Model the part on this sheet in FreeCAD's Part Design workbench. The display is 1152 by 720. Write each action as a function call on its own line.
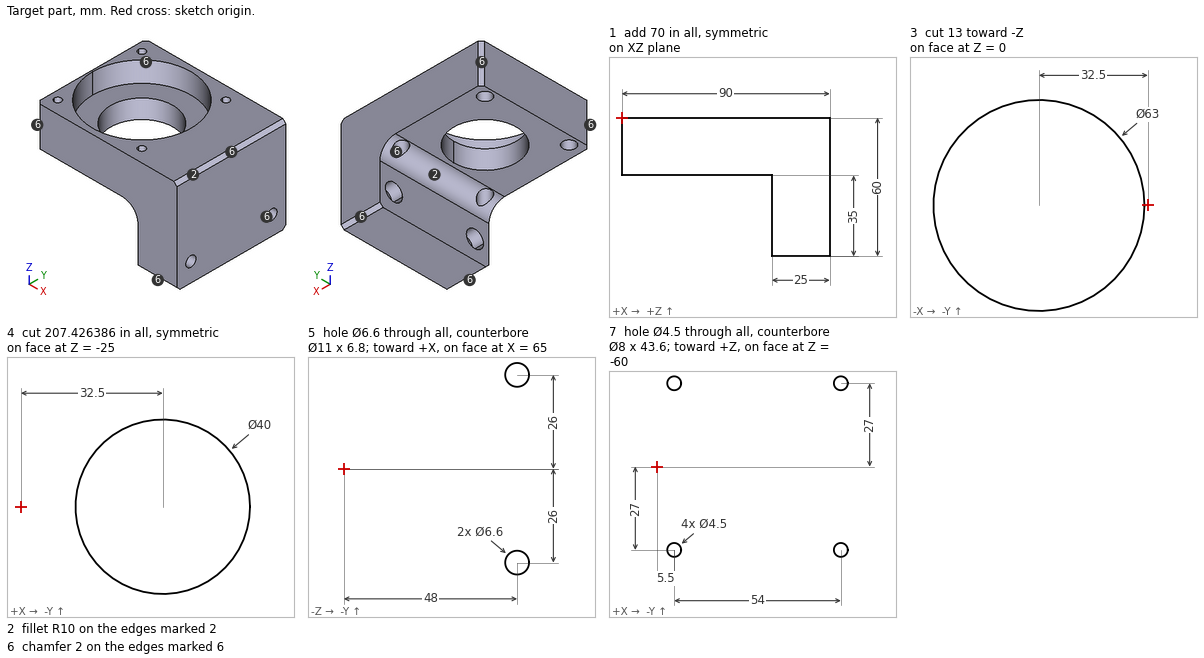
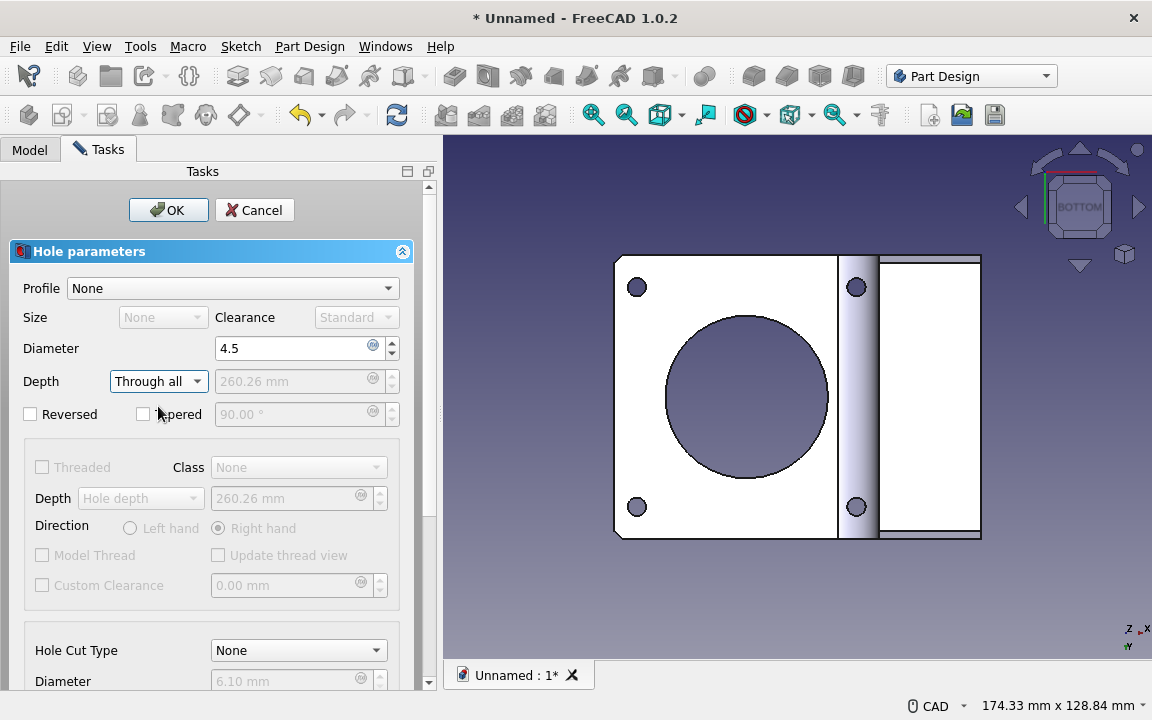
click(300, 650)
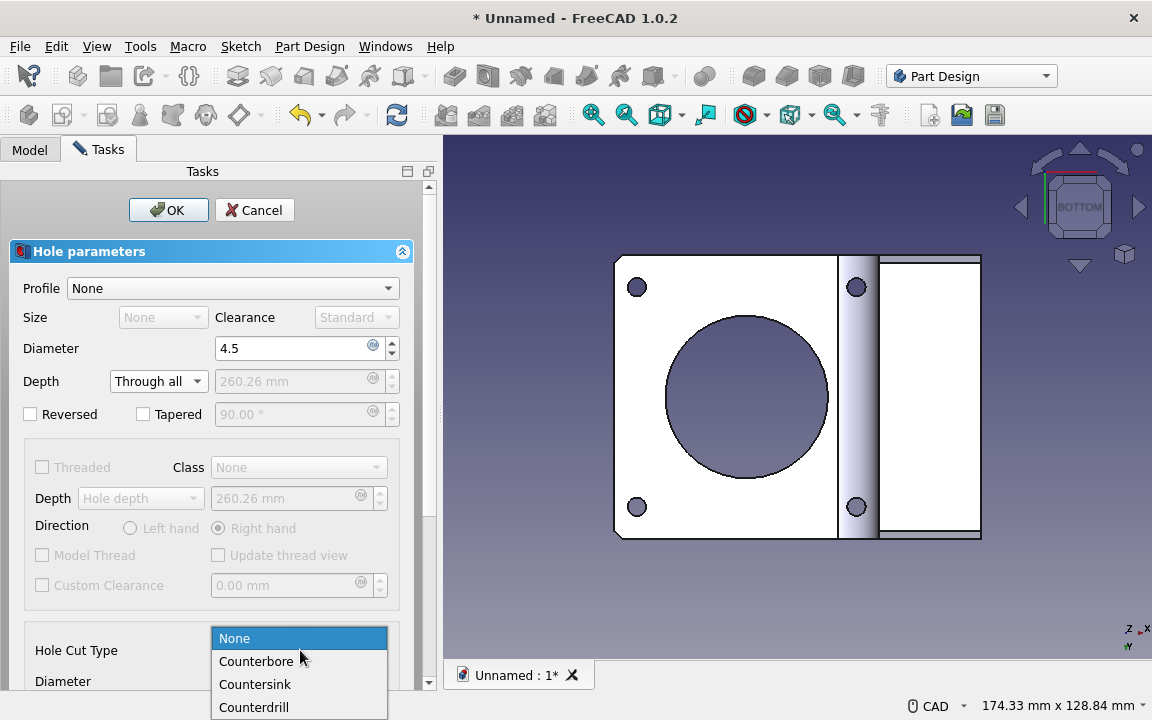
click(298, 662)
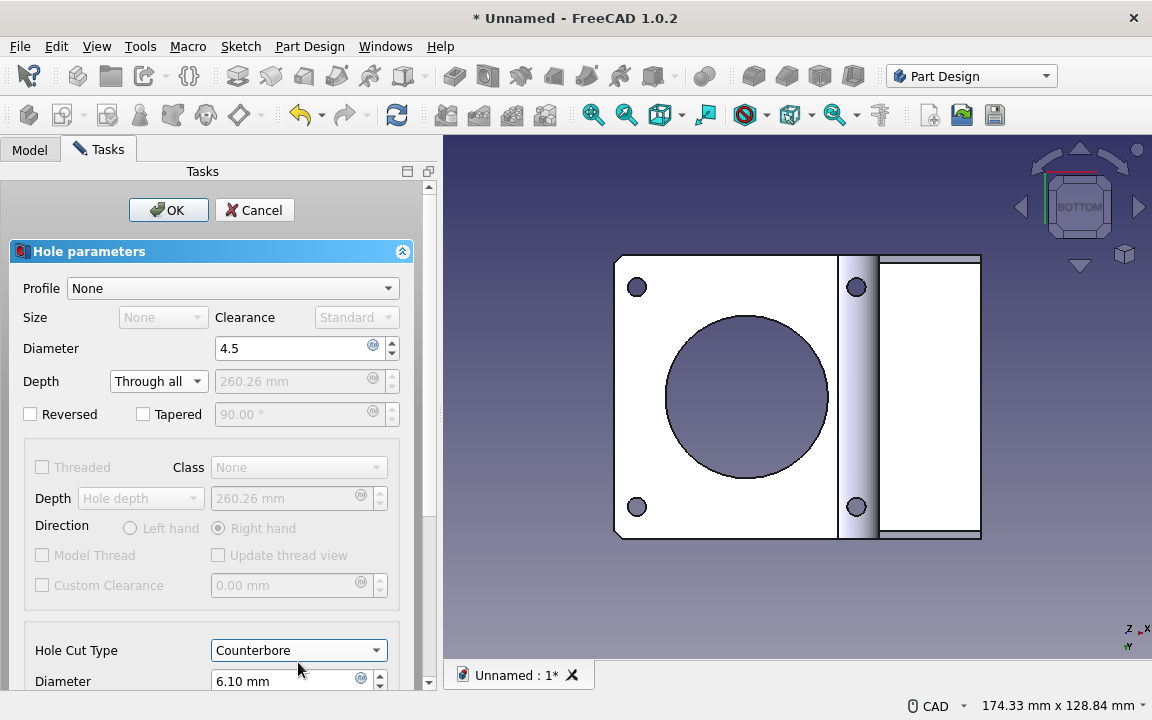
scroll(429, 436, down, 2)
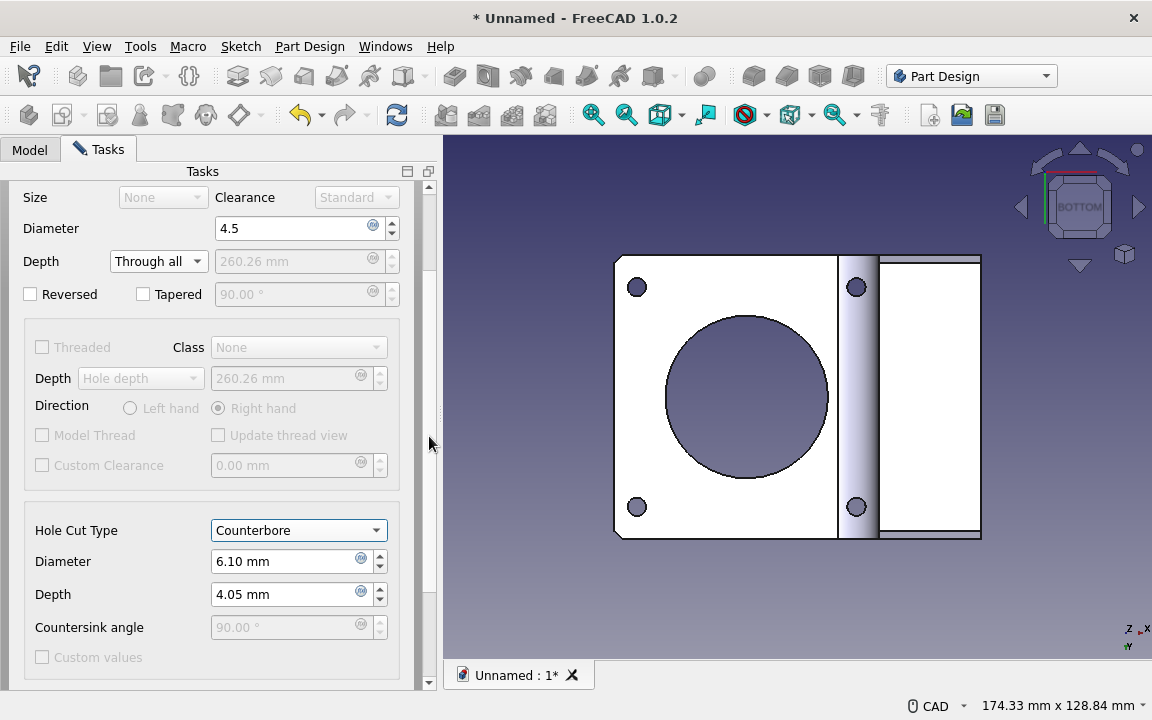
triple_click(292, 562)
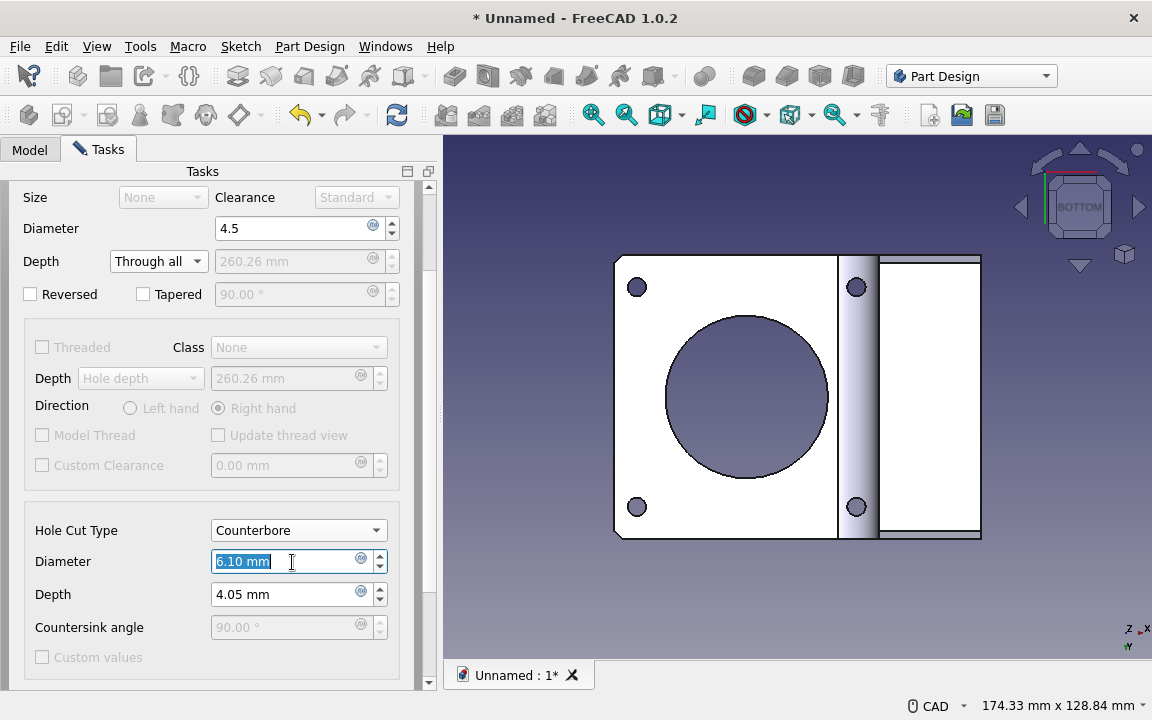
text(8)
key(Tab)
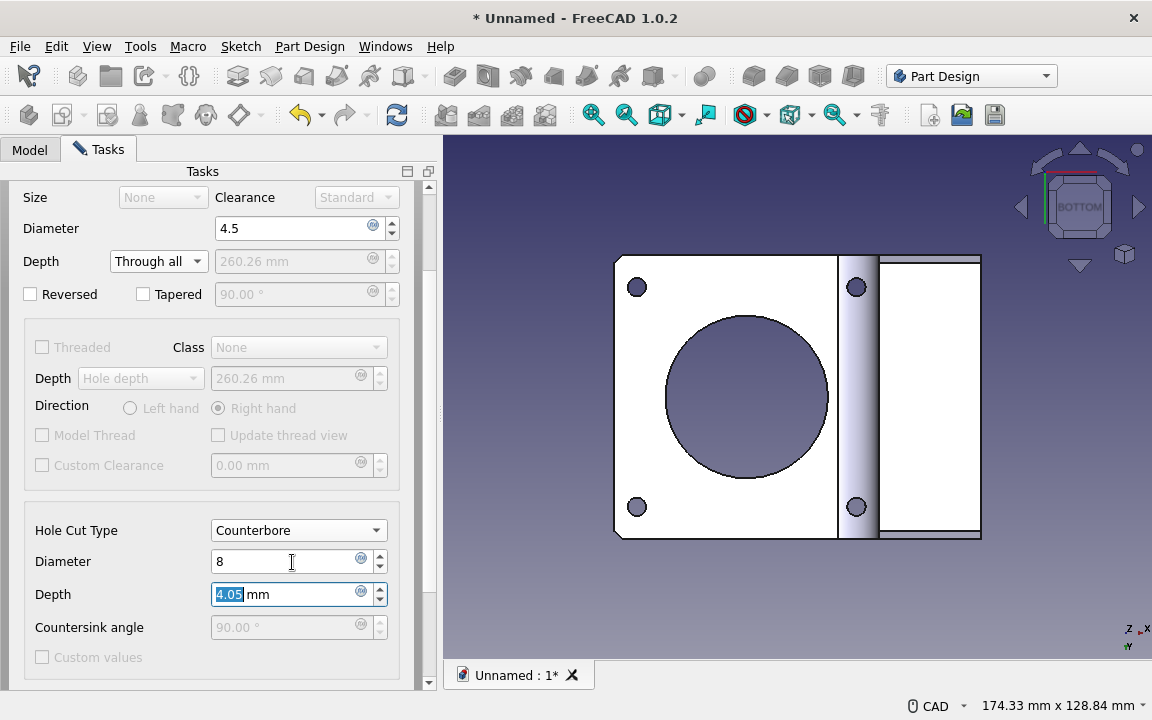
text(43.6)
key(Tab)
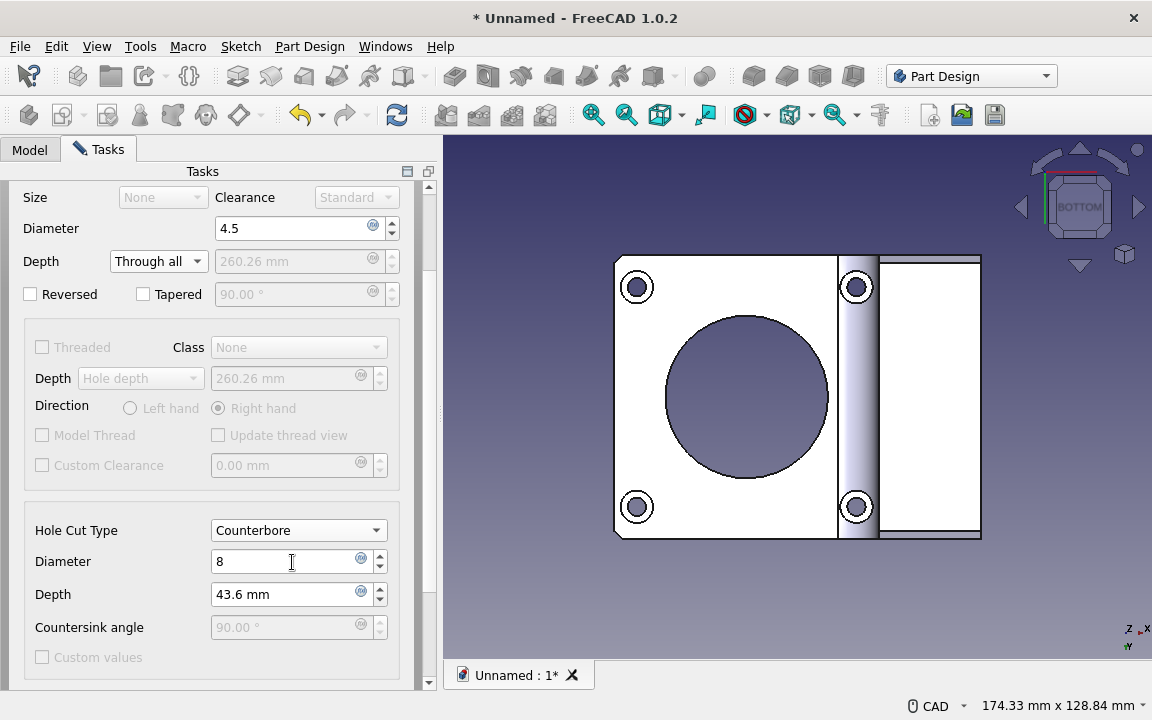
scroll(429, 436, up, 3)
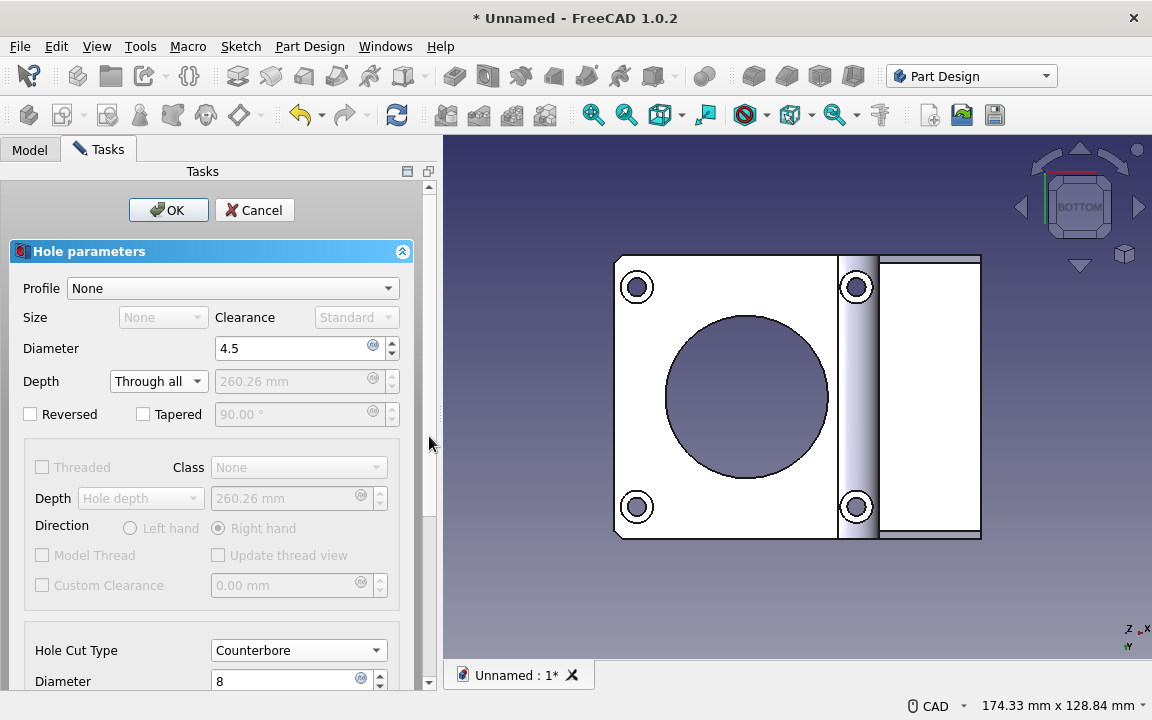
click(169, 210)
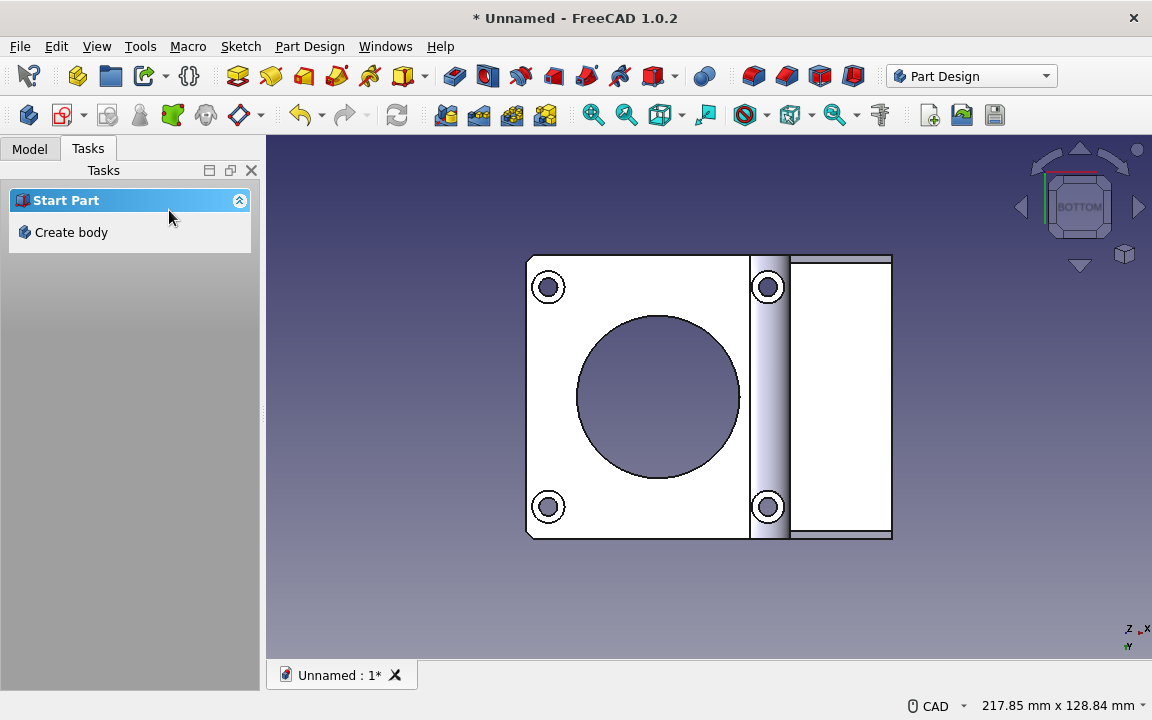
key(0)